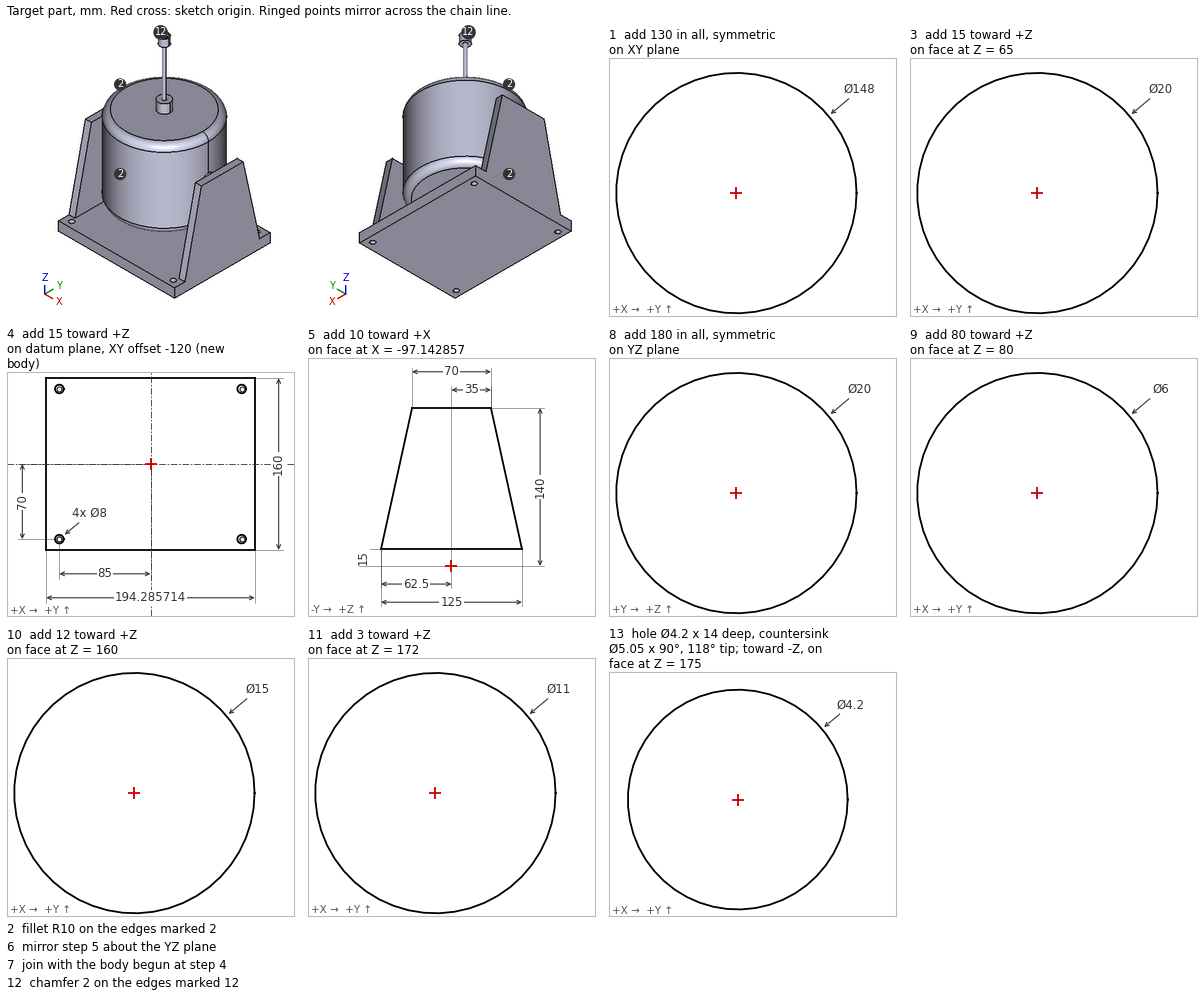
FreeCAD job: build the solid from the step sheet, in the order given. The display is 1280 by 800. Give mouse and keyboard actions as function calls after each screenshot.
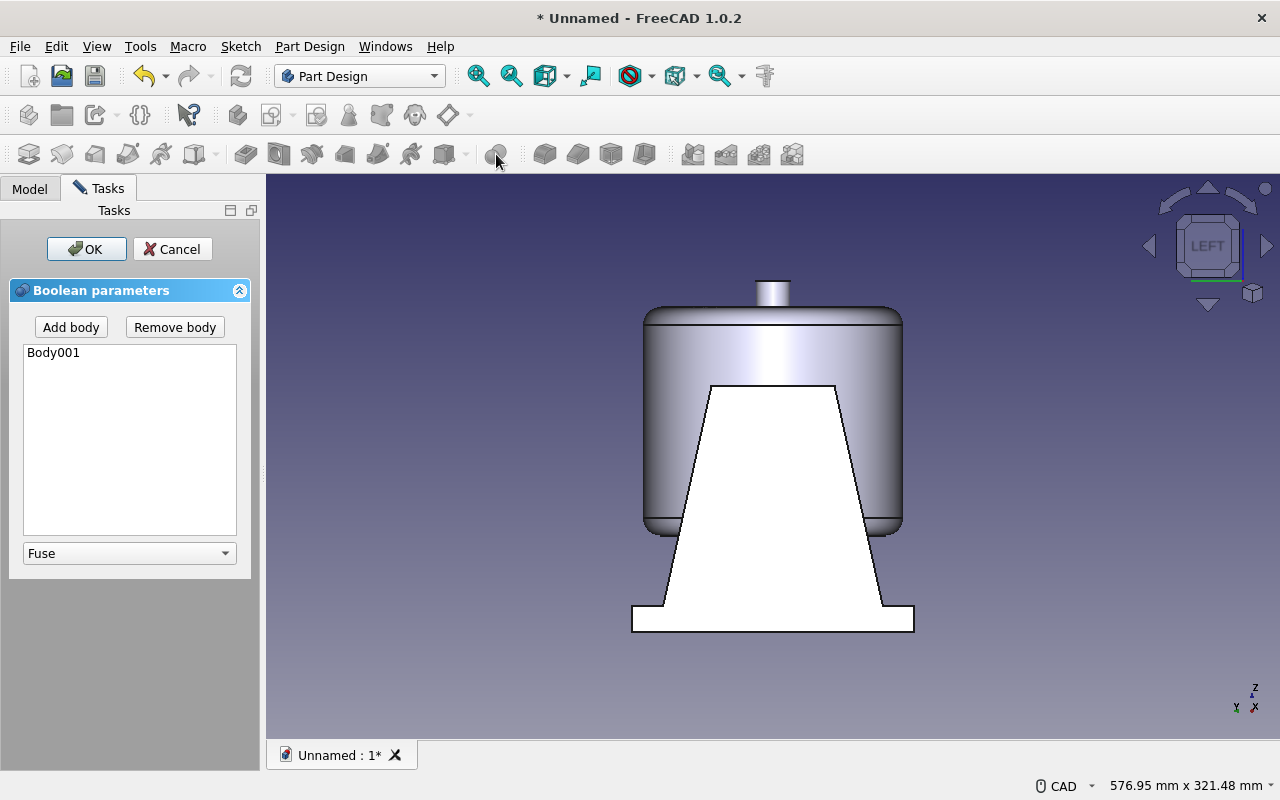
click(87, 249)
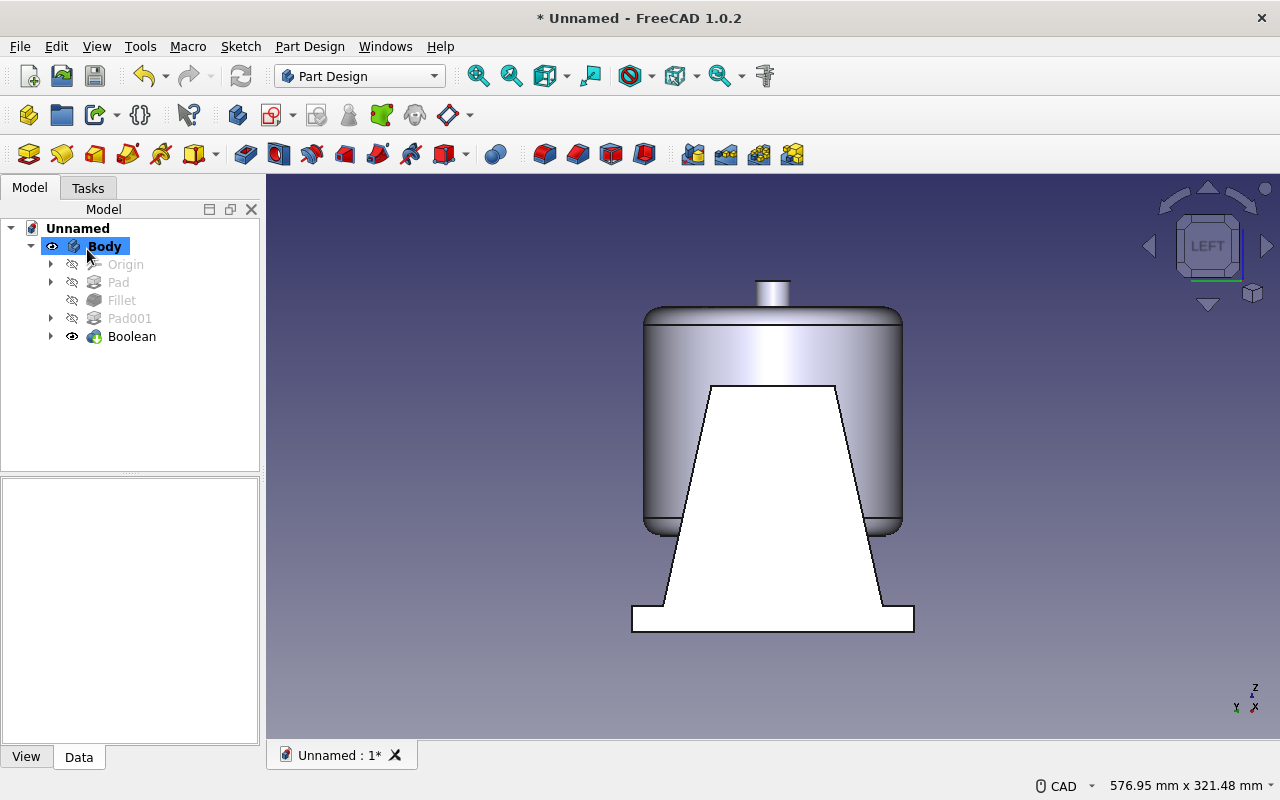
click(270, 116)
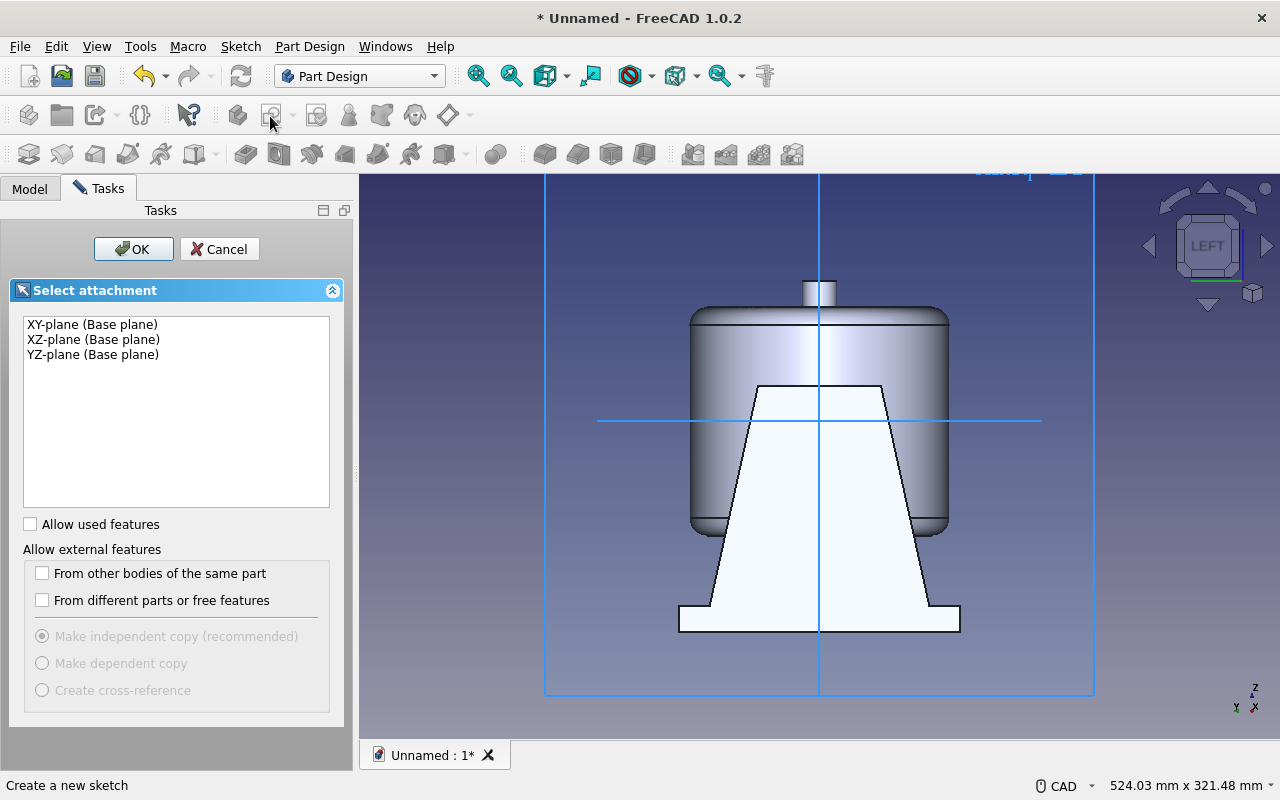
click(84, 354)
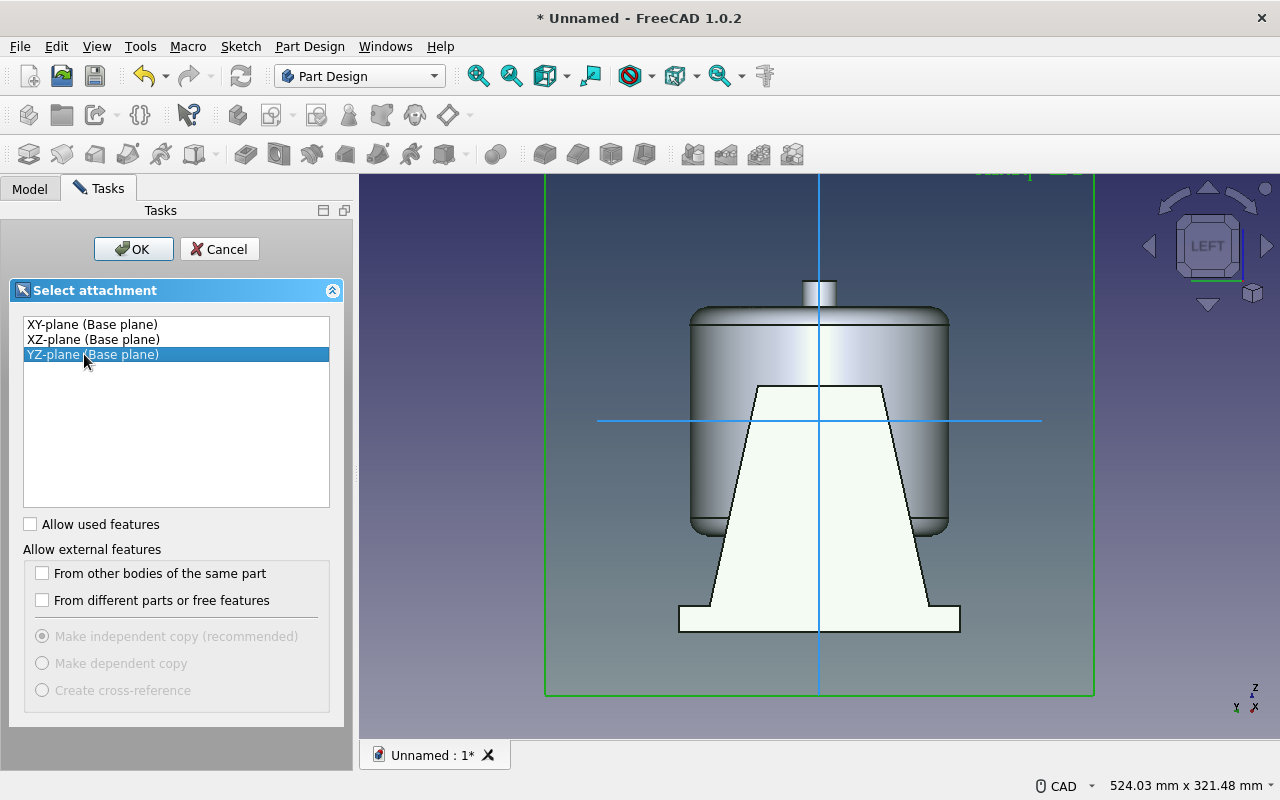
click(134, 249)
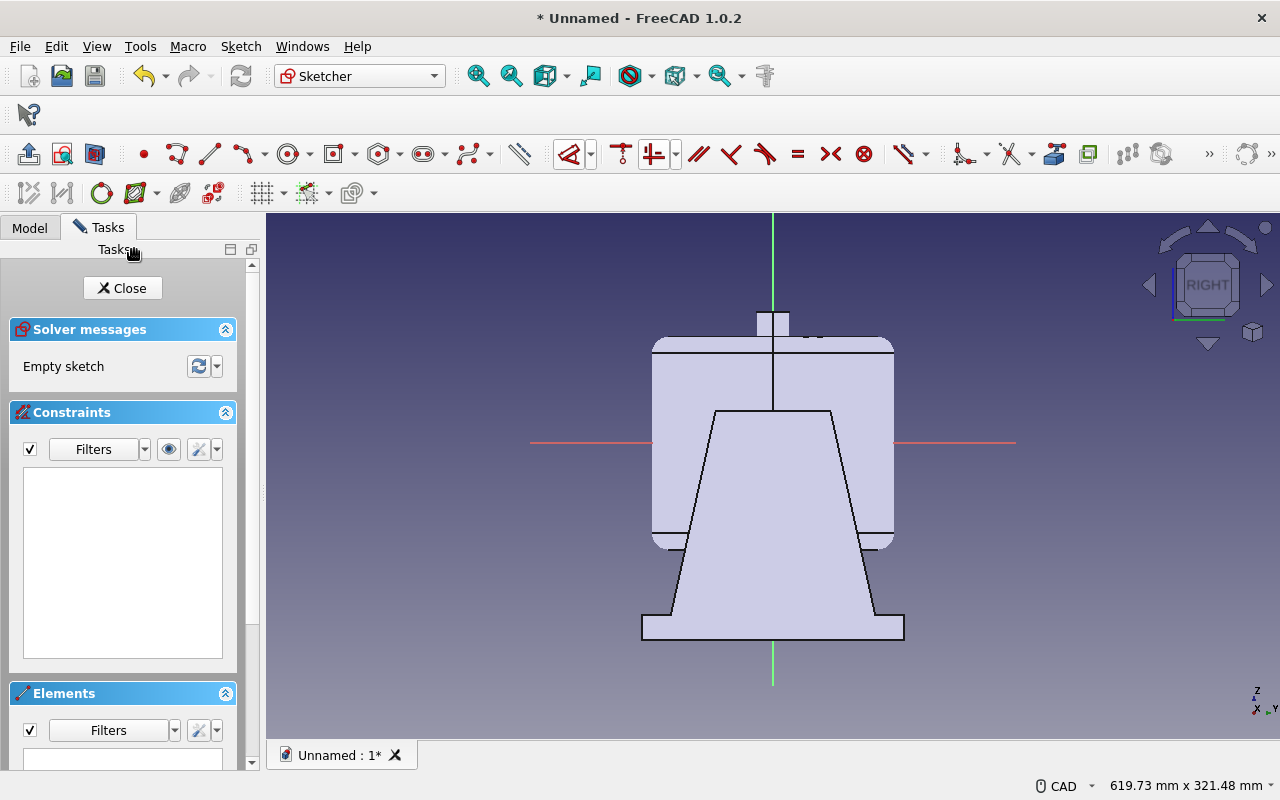
key(q)
key(s)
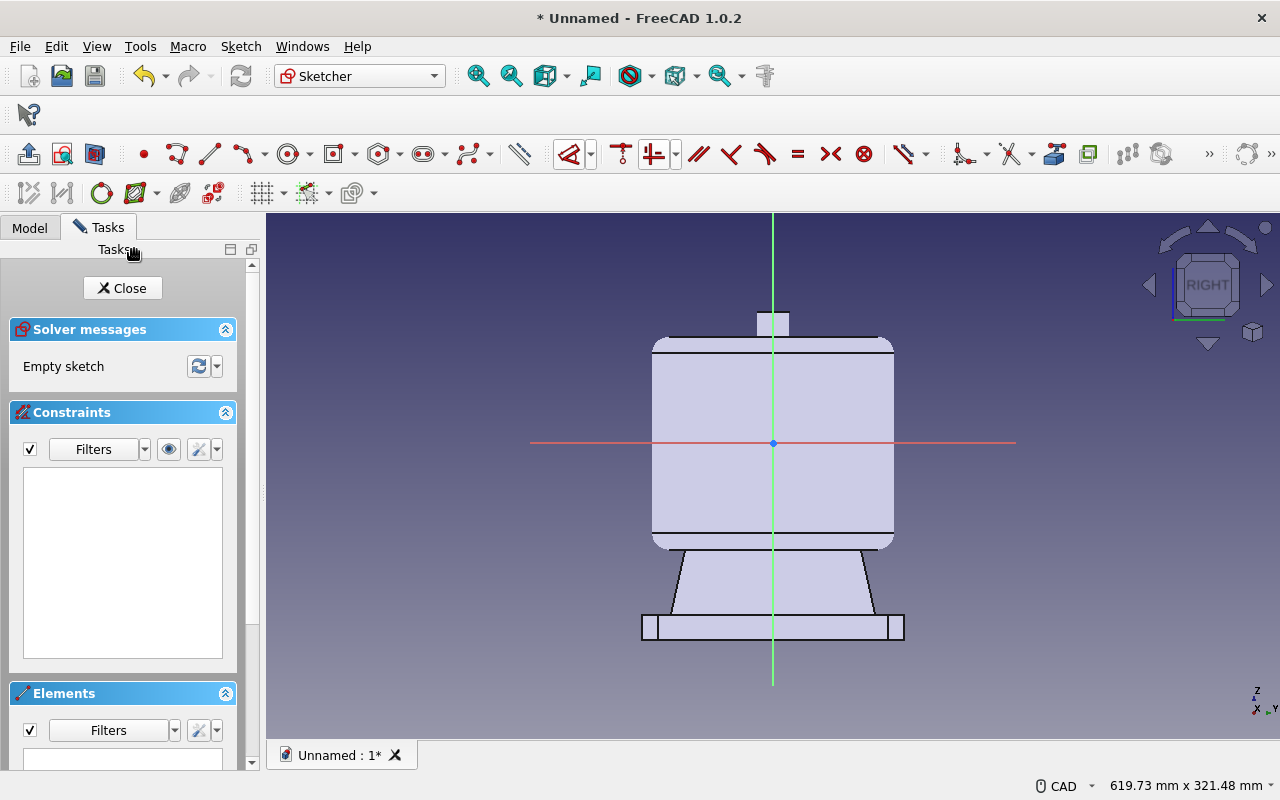
scroll(780, 440, up, 12)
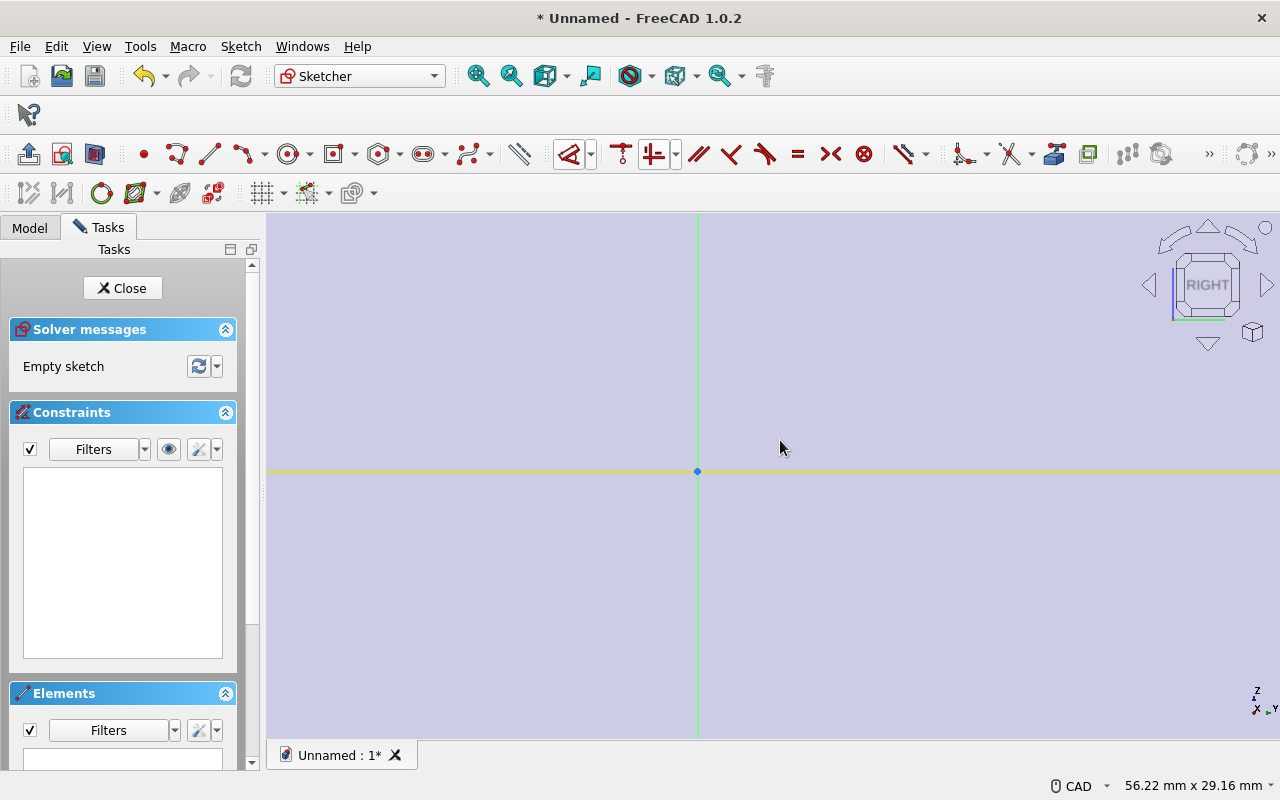
click(288, 154)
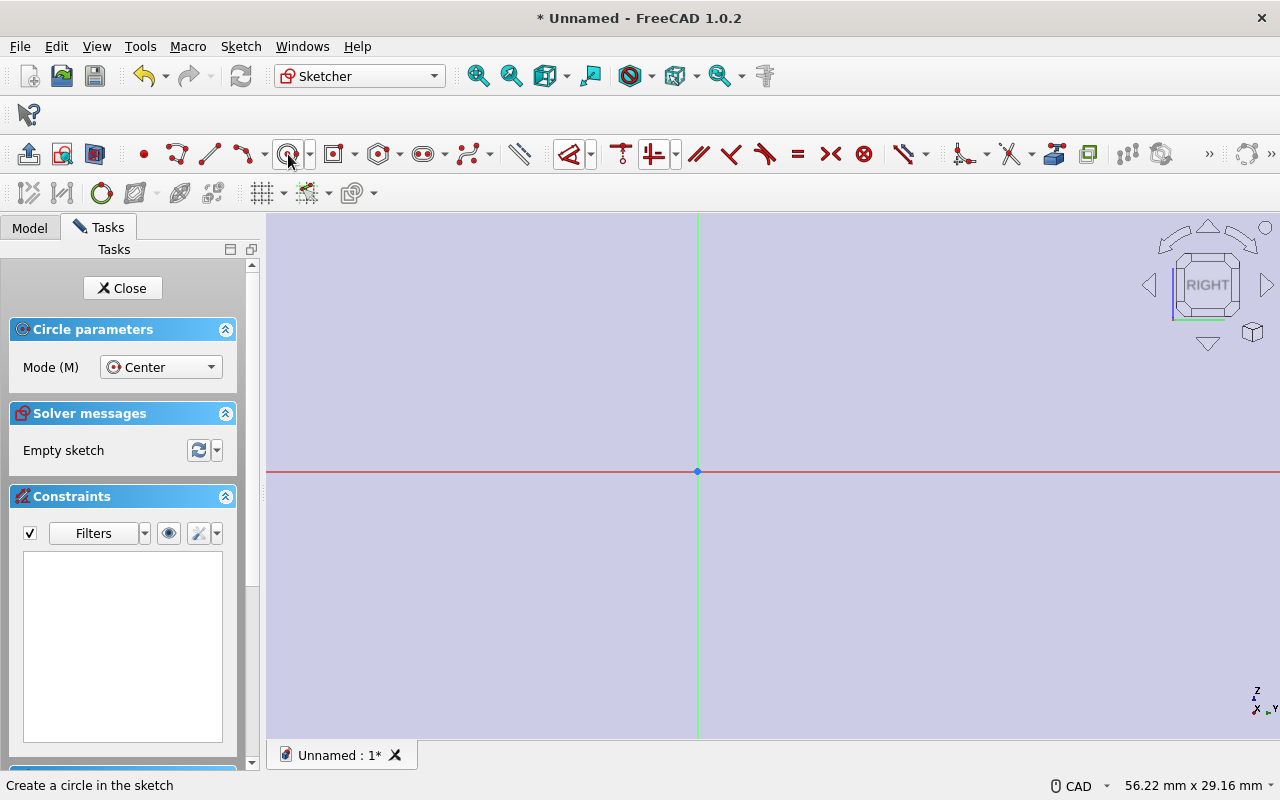
click(698, 472)
click(825, 344)
key(Escape)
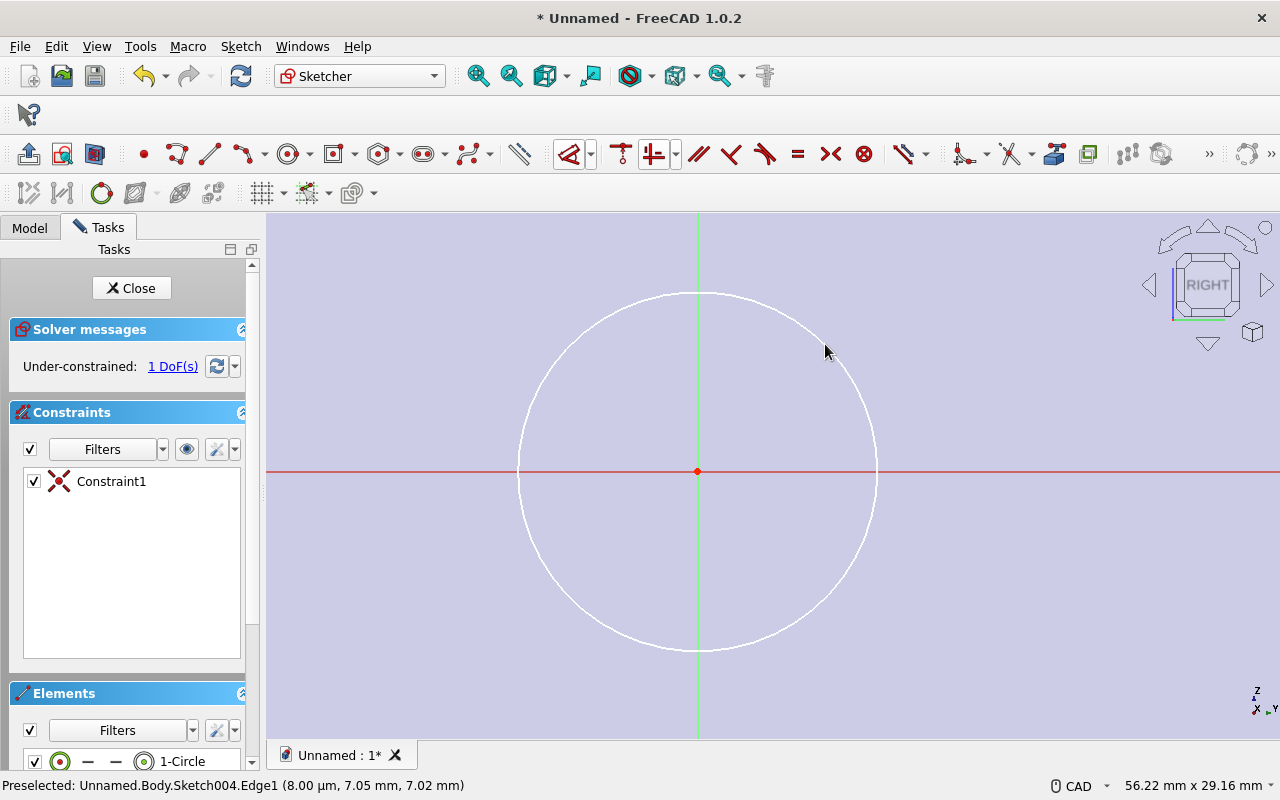
click(824, 344)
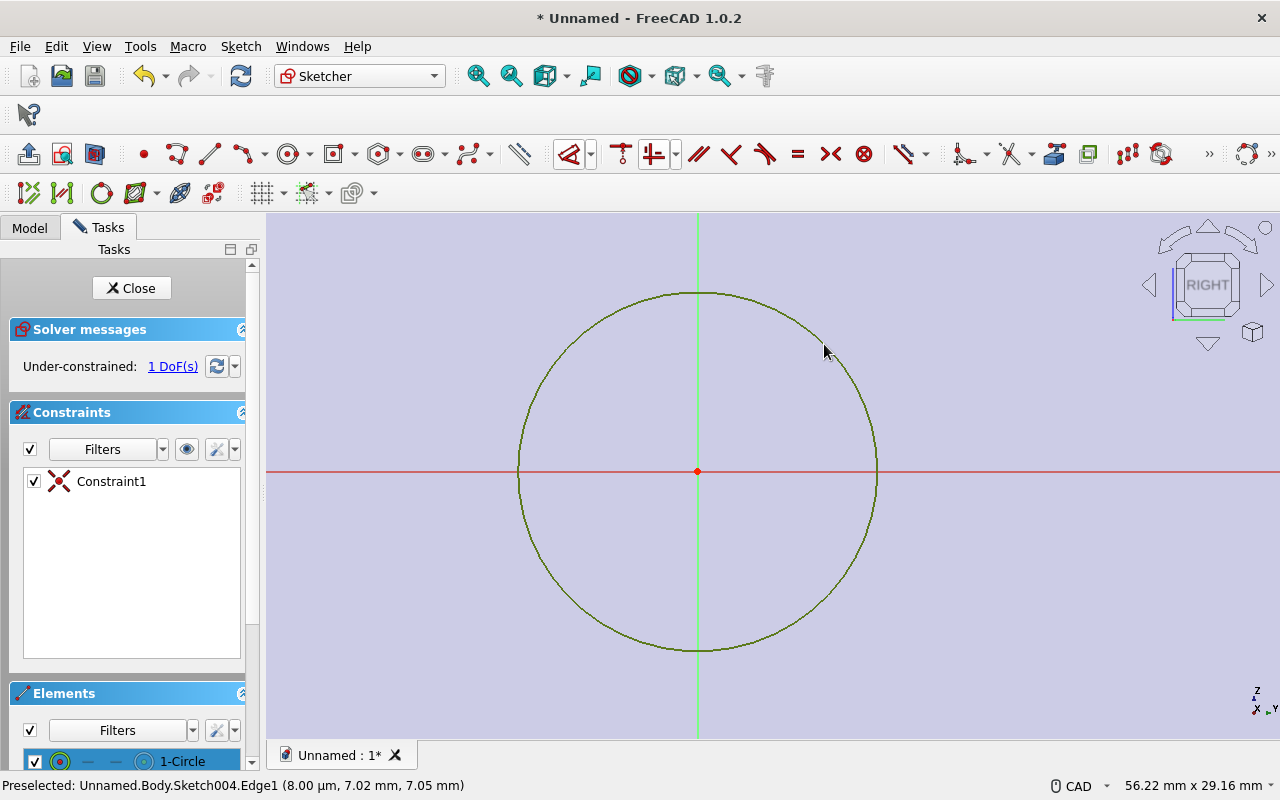
key(k)
key(o)